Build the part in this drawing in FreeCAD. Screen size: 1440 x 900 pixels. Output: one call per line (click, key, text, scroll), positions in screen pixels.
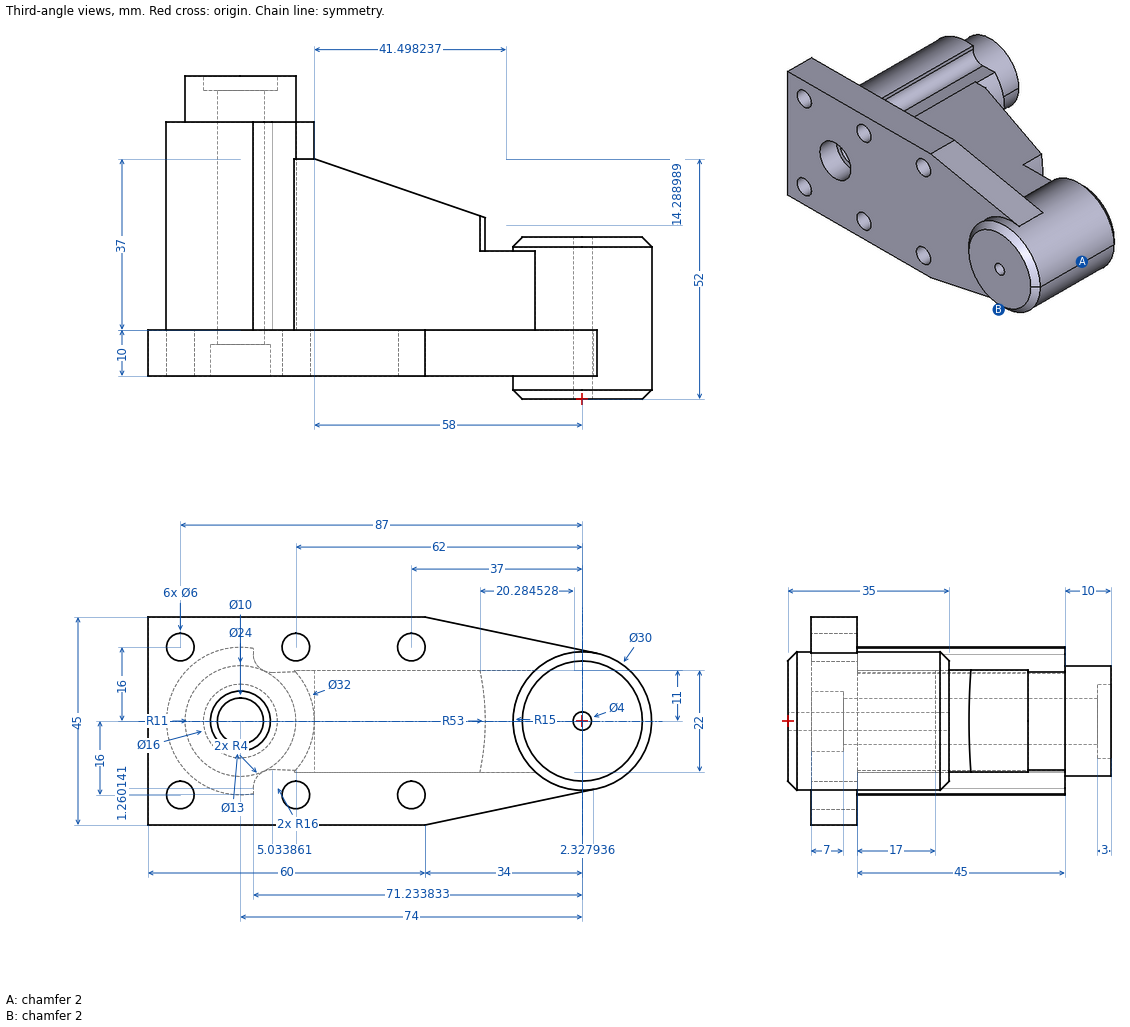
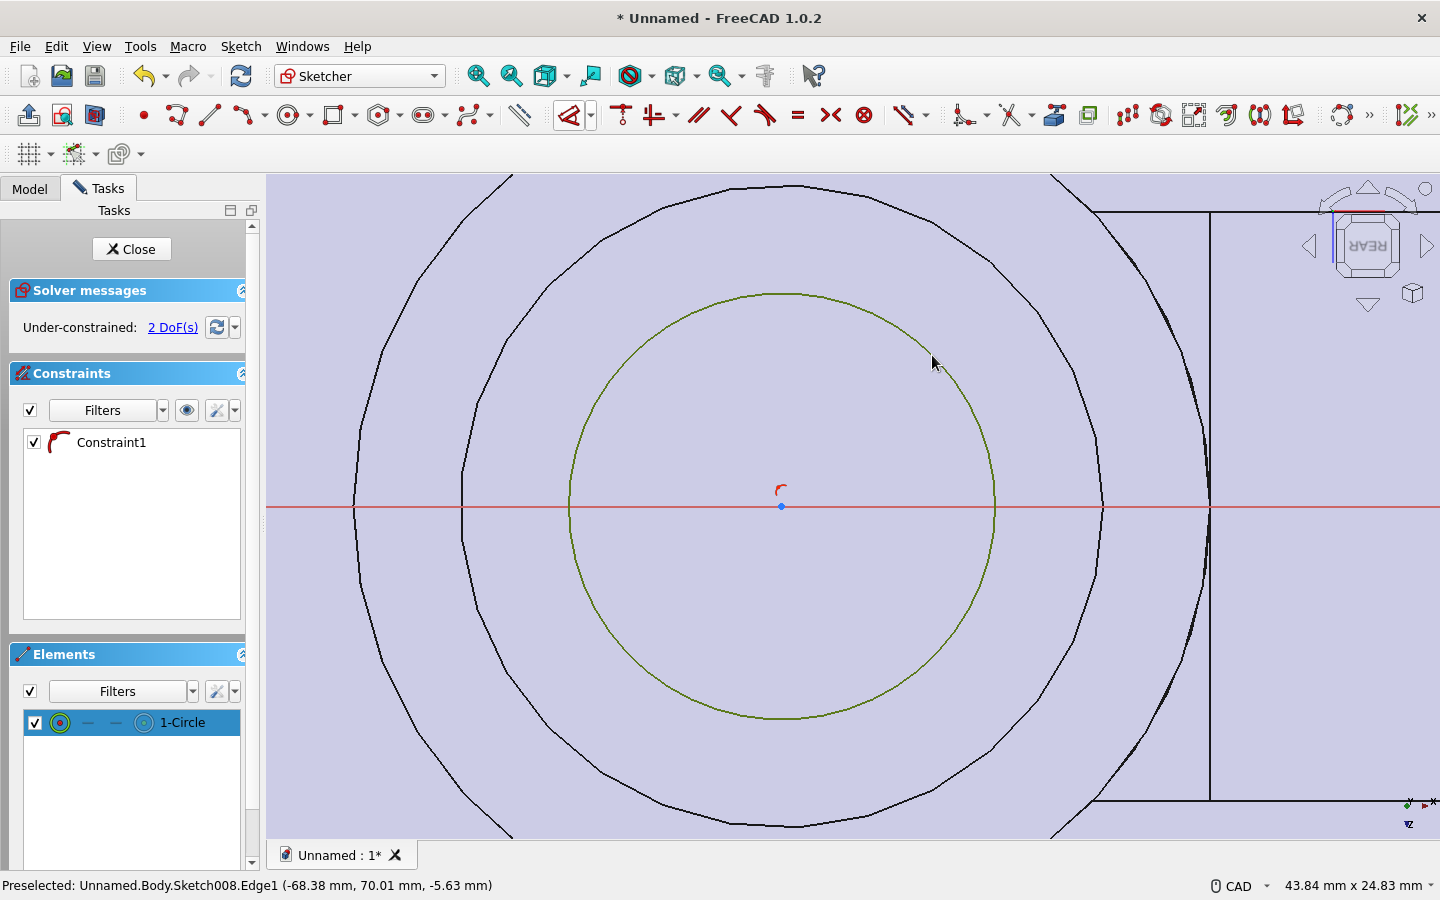
click(590, 116)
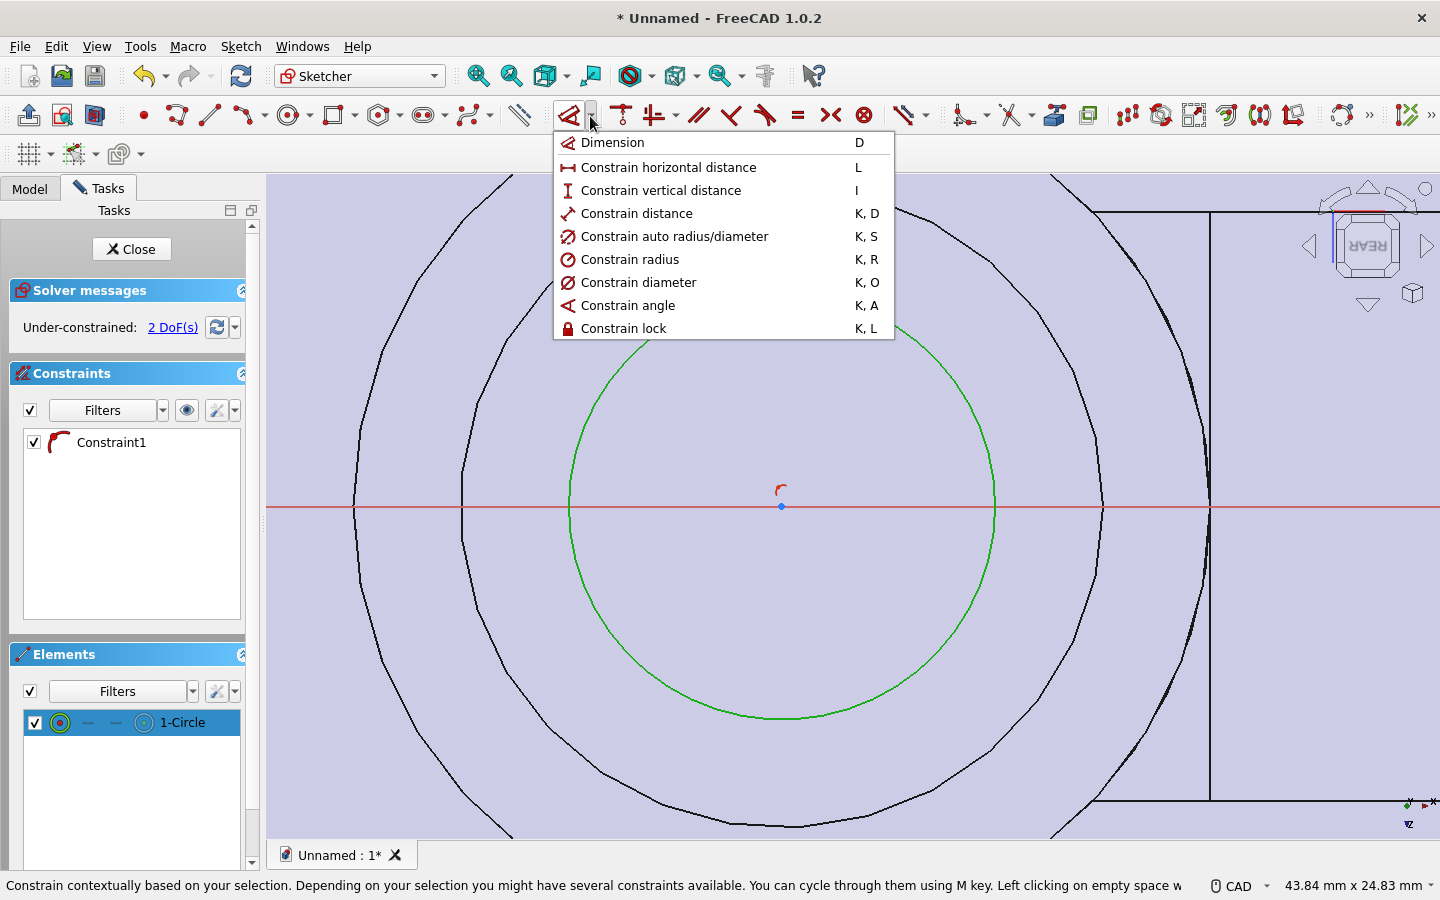
click(724, 282)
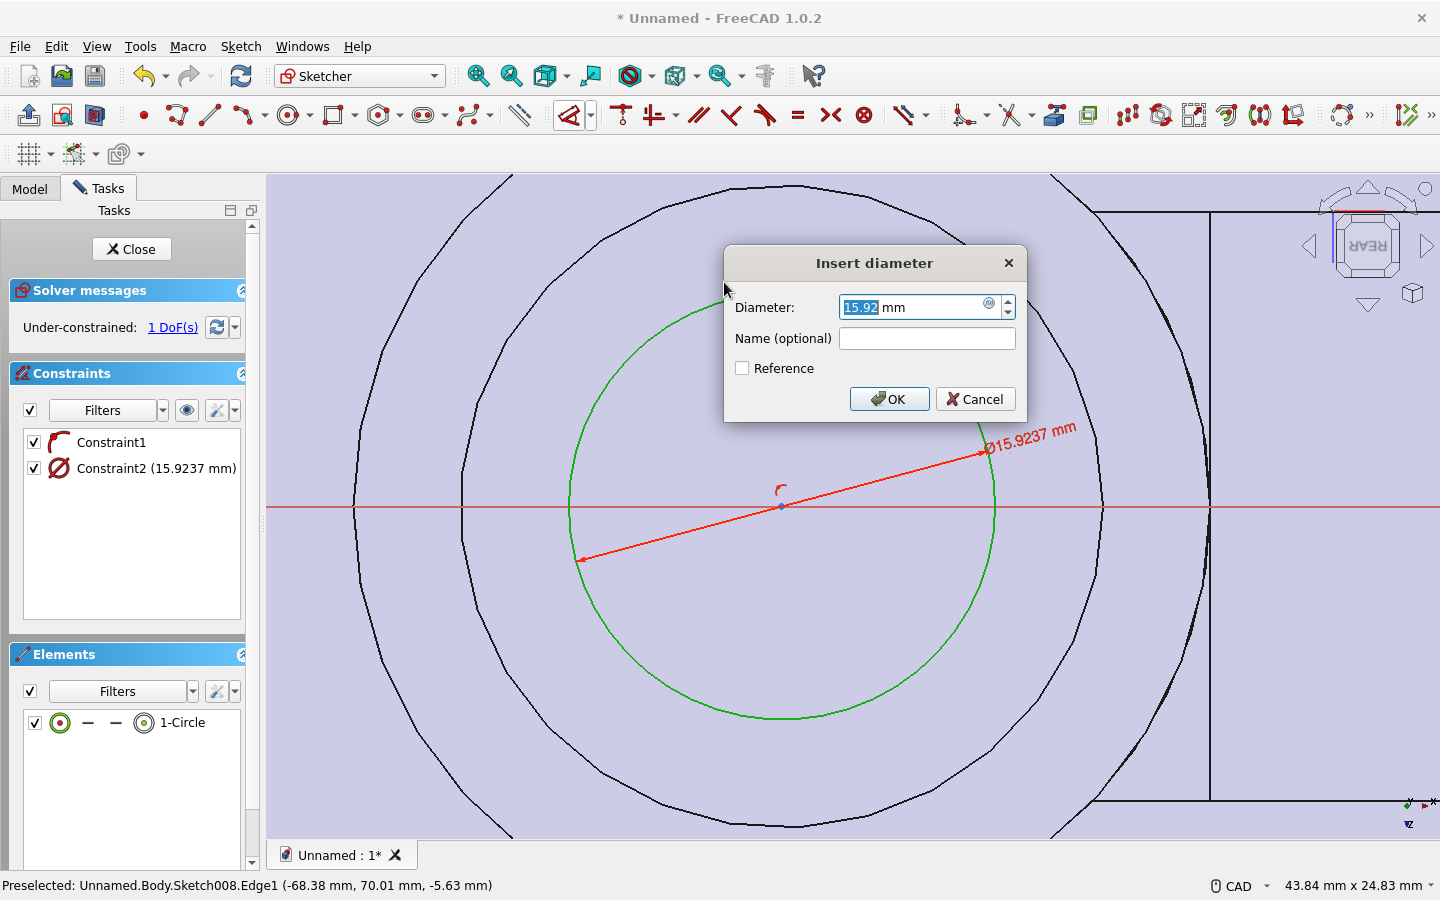
text(16)
key(Return)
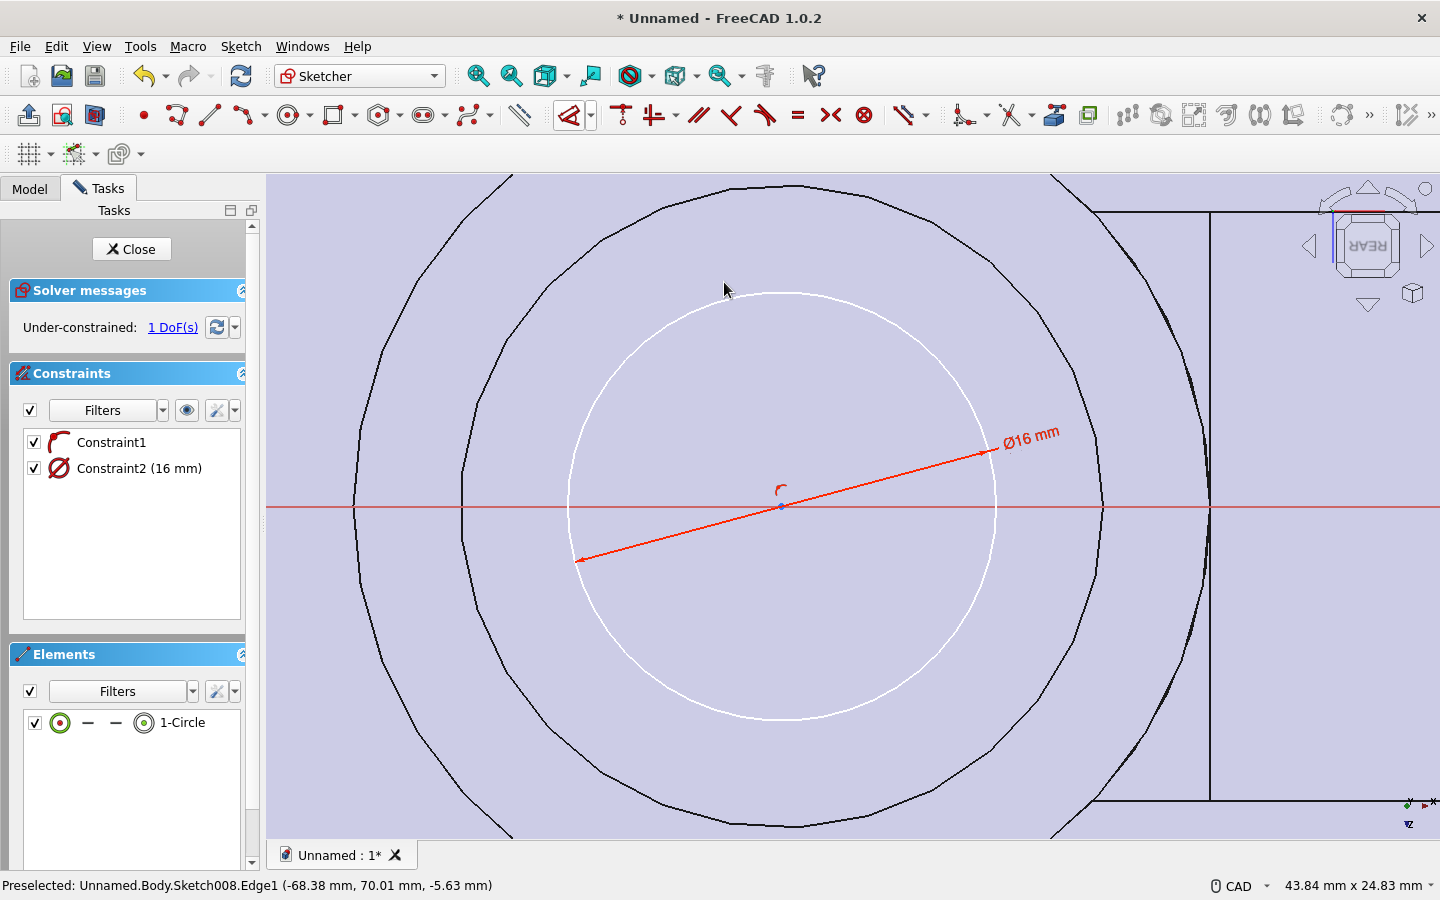
click(782, 506)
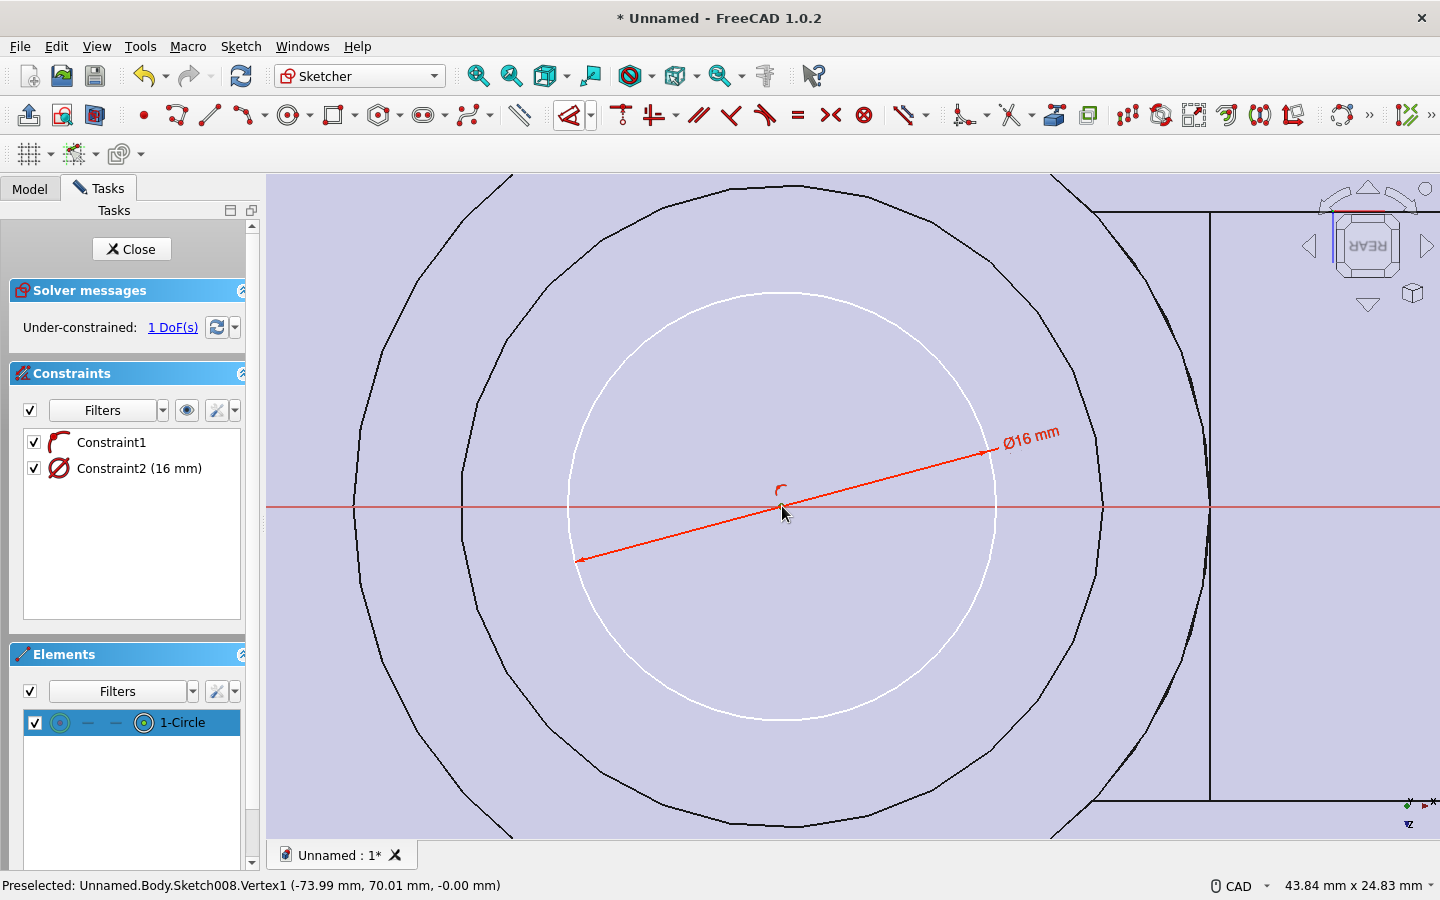
click(590, 116)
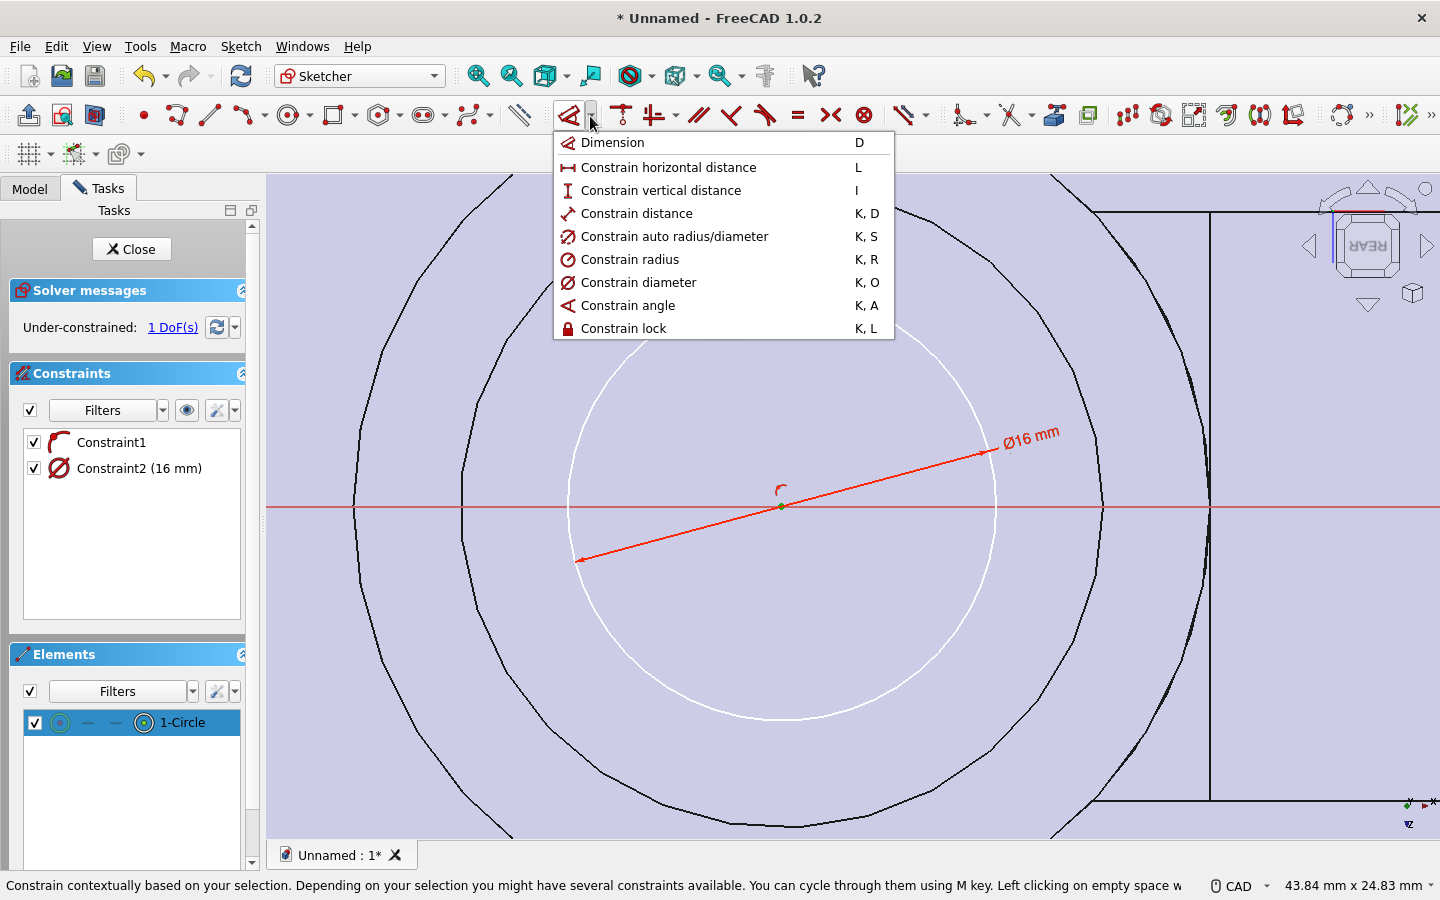
click(724, 168)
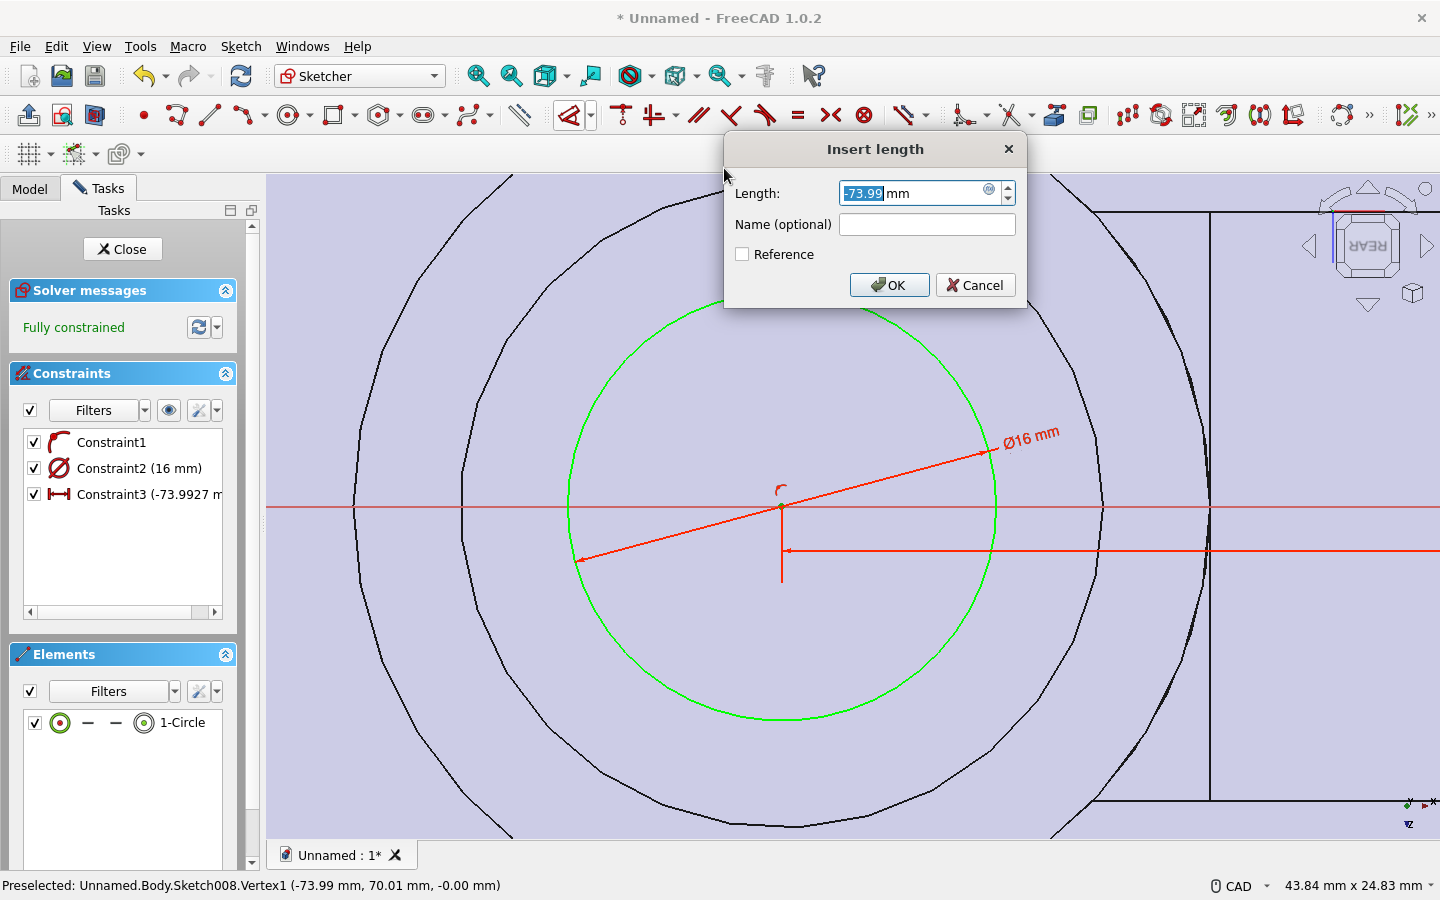
text(-74)
key(Return)